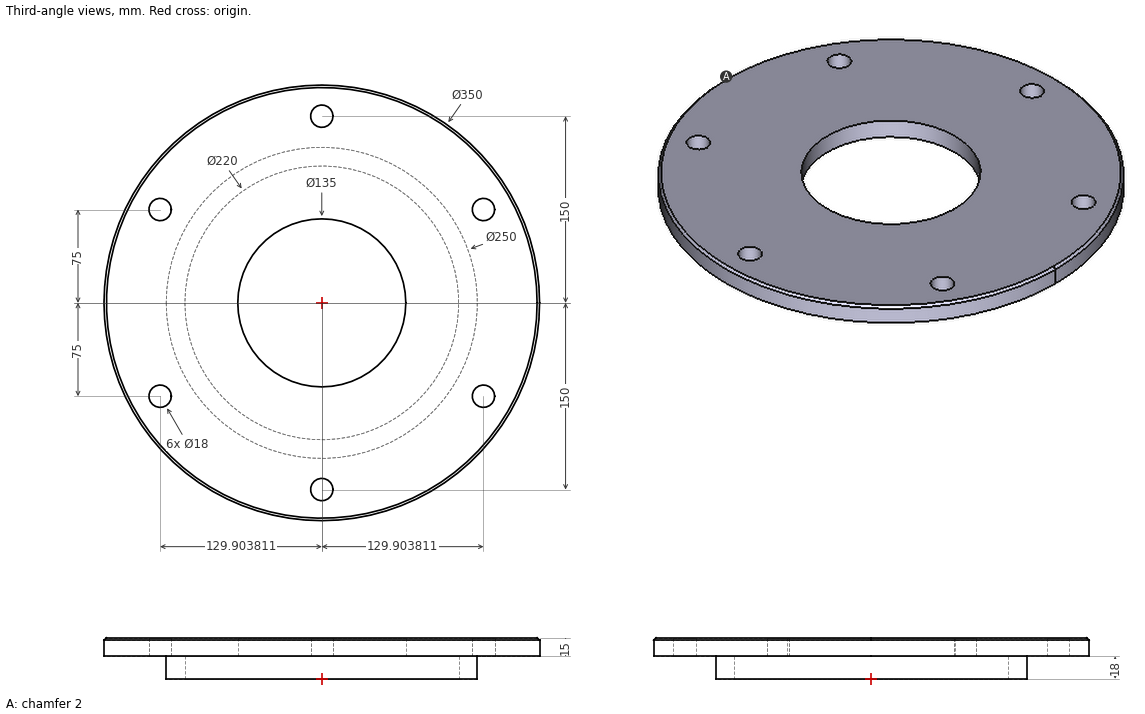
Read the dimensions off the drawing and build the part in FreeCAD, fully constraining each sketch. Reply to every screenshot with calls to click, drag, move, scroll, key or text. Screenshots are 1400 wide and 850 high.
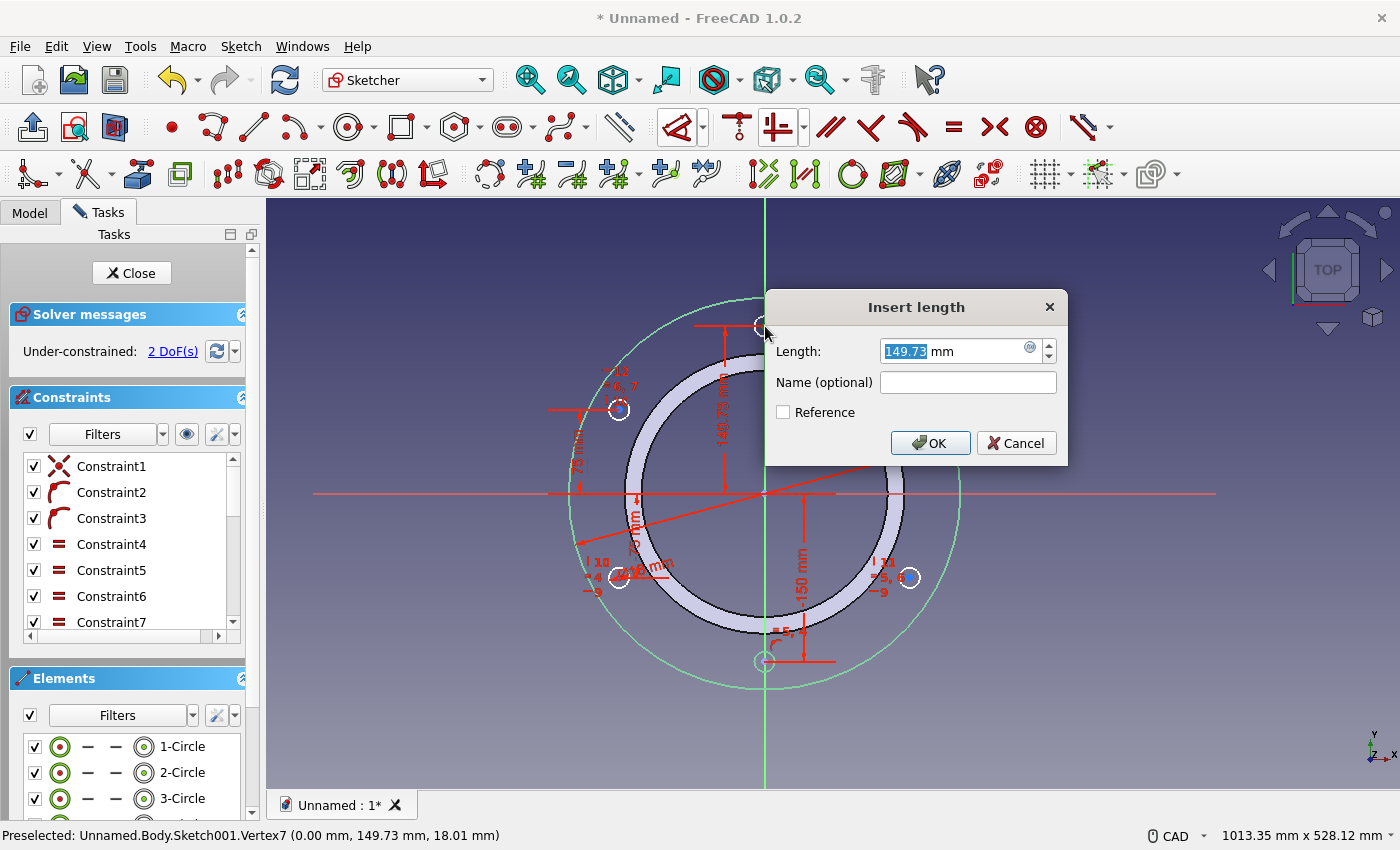
text(150)
key(Return)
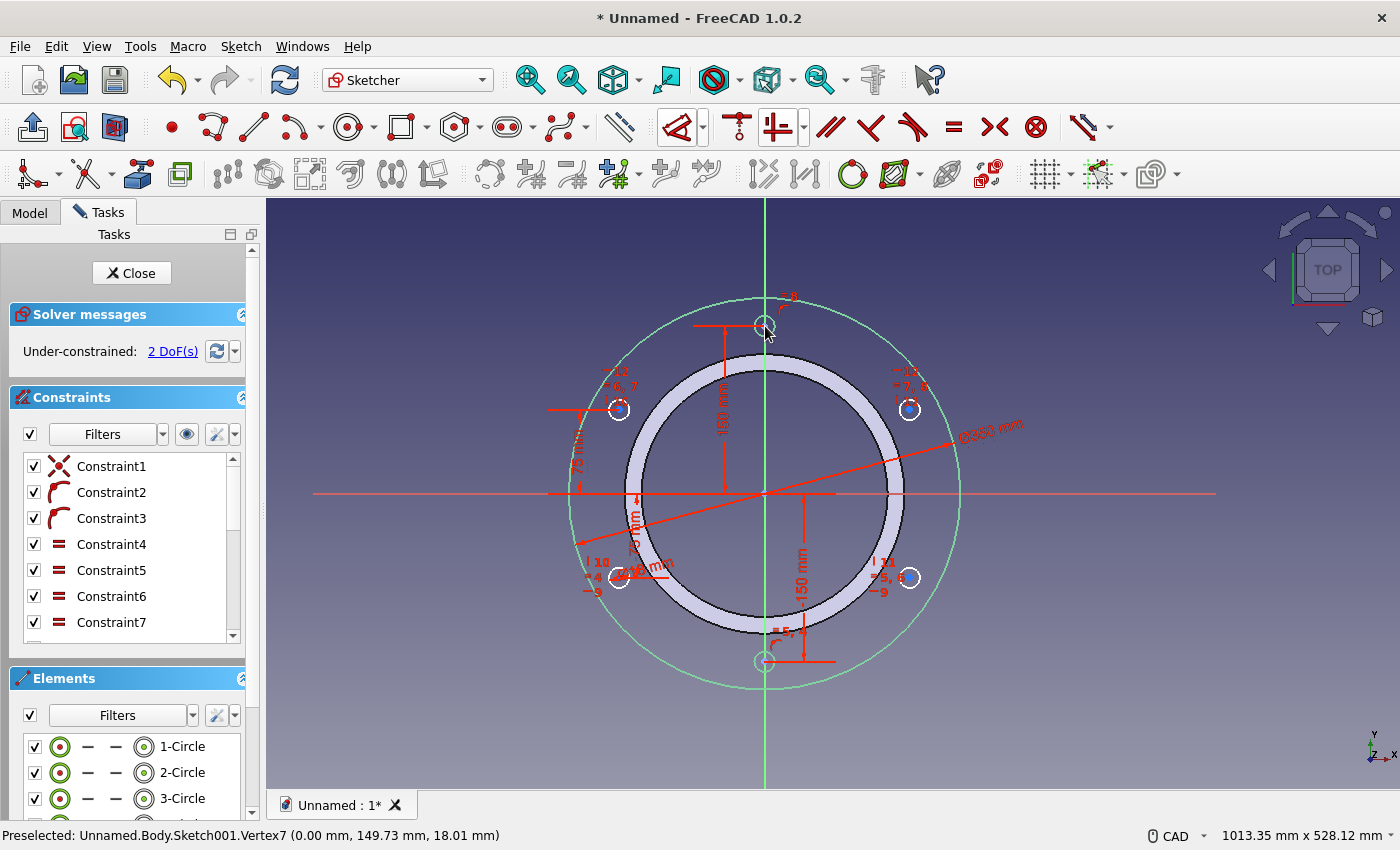
click(619, 578)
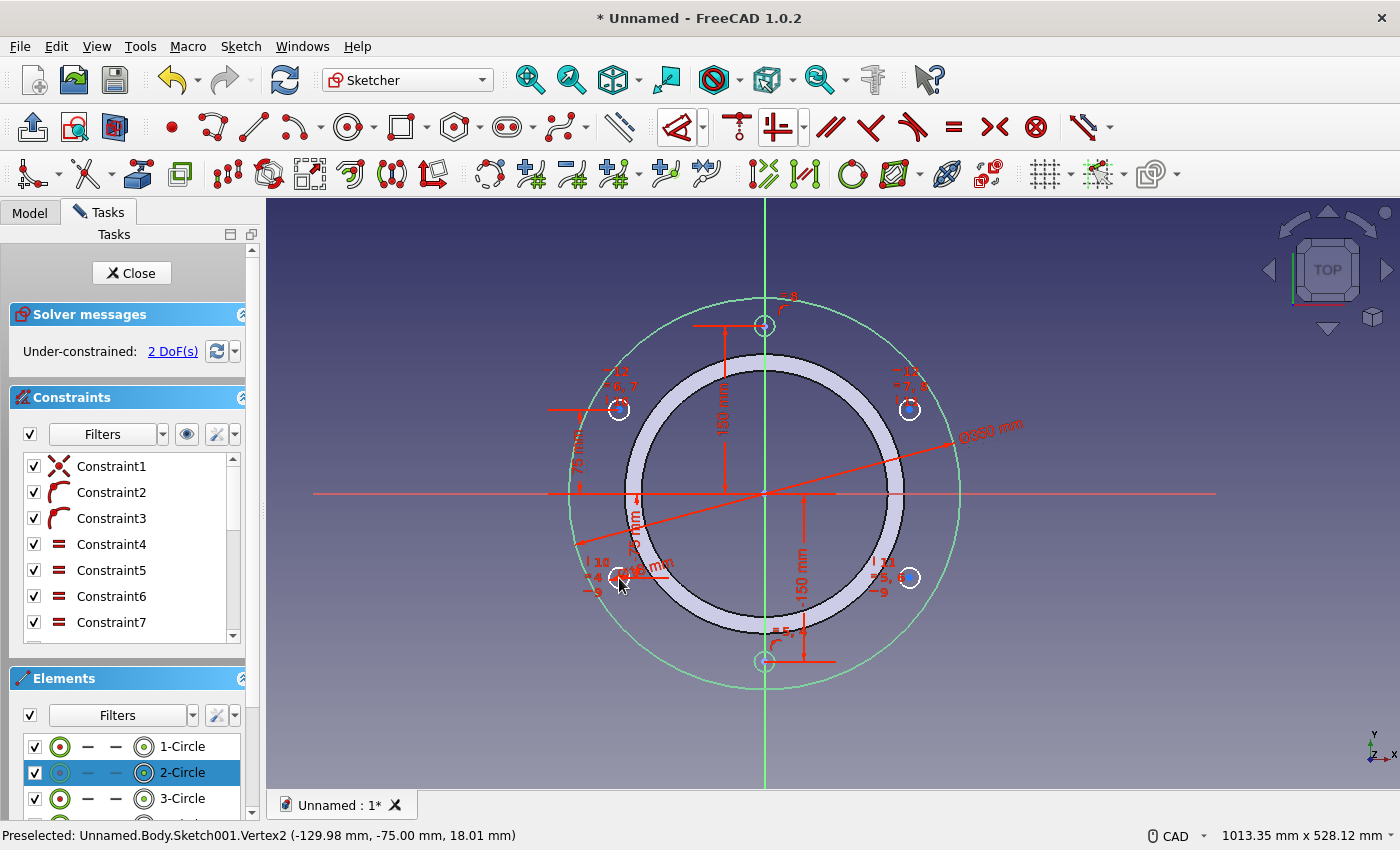
click(702, 128)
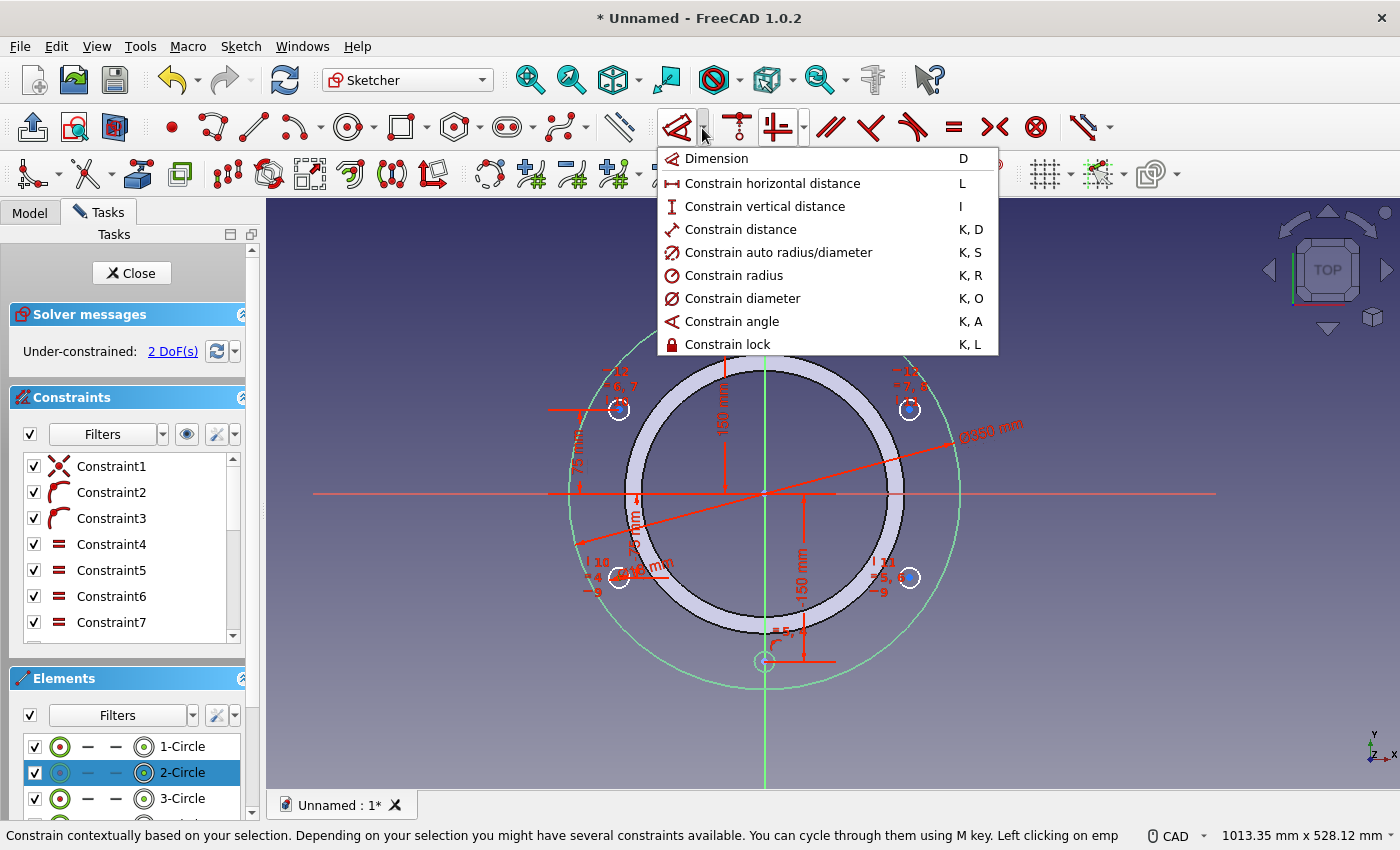
click(828, 184)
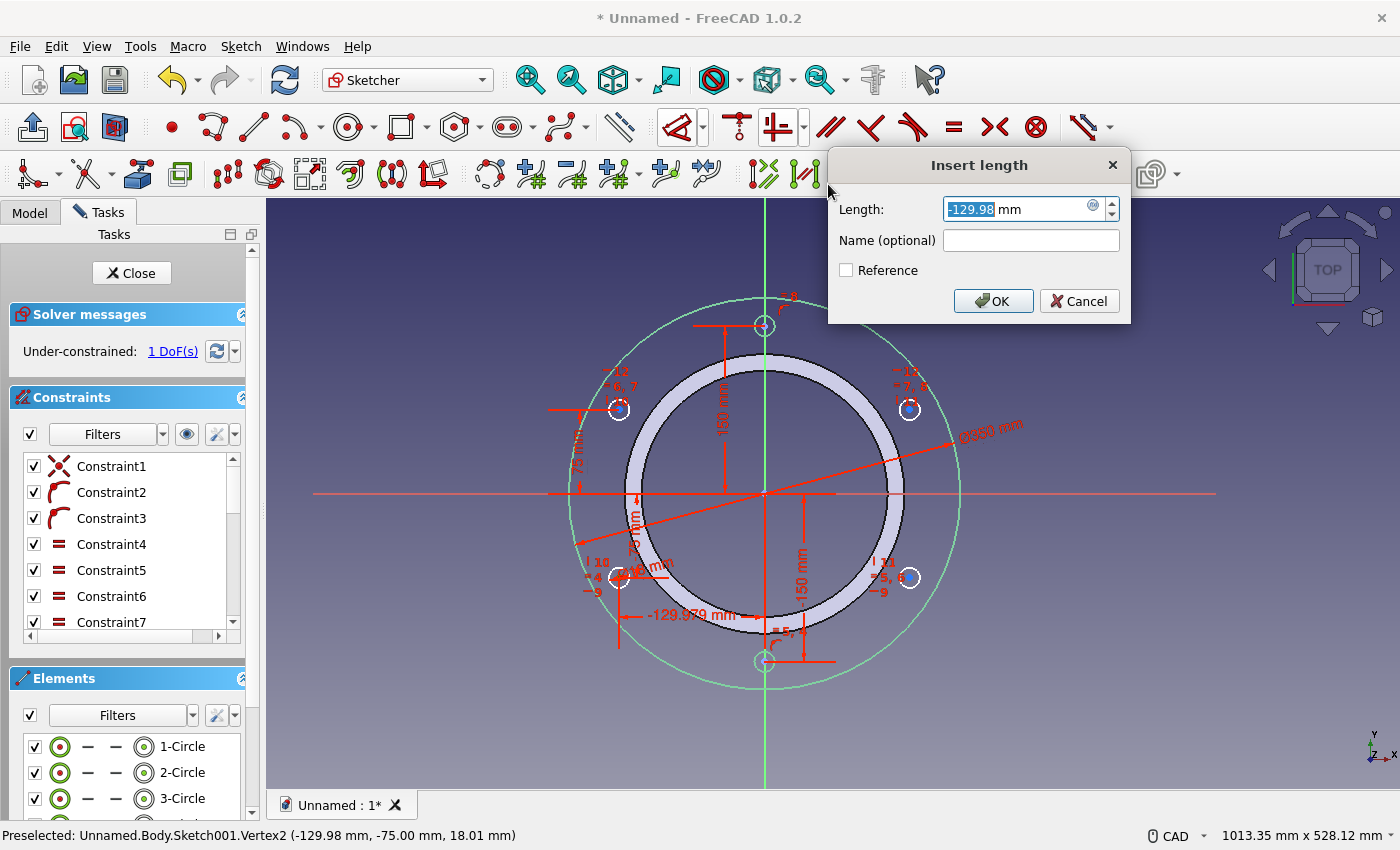
text(-129.903811)
key(Return)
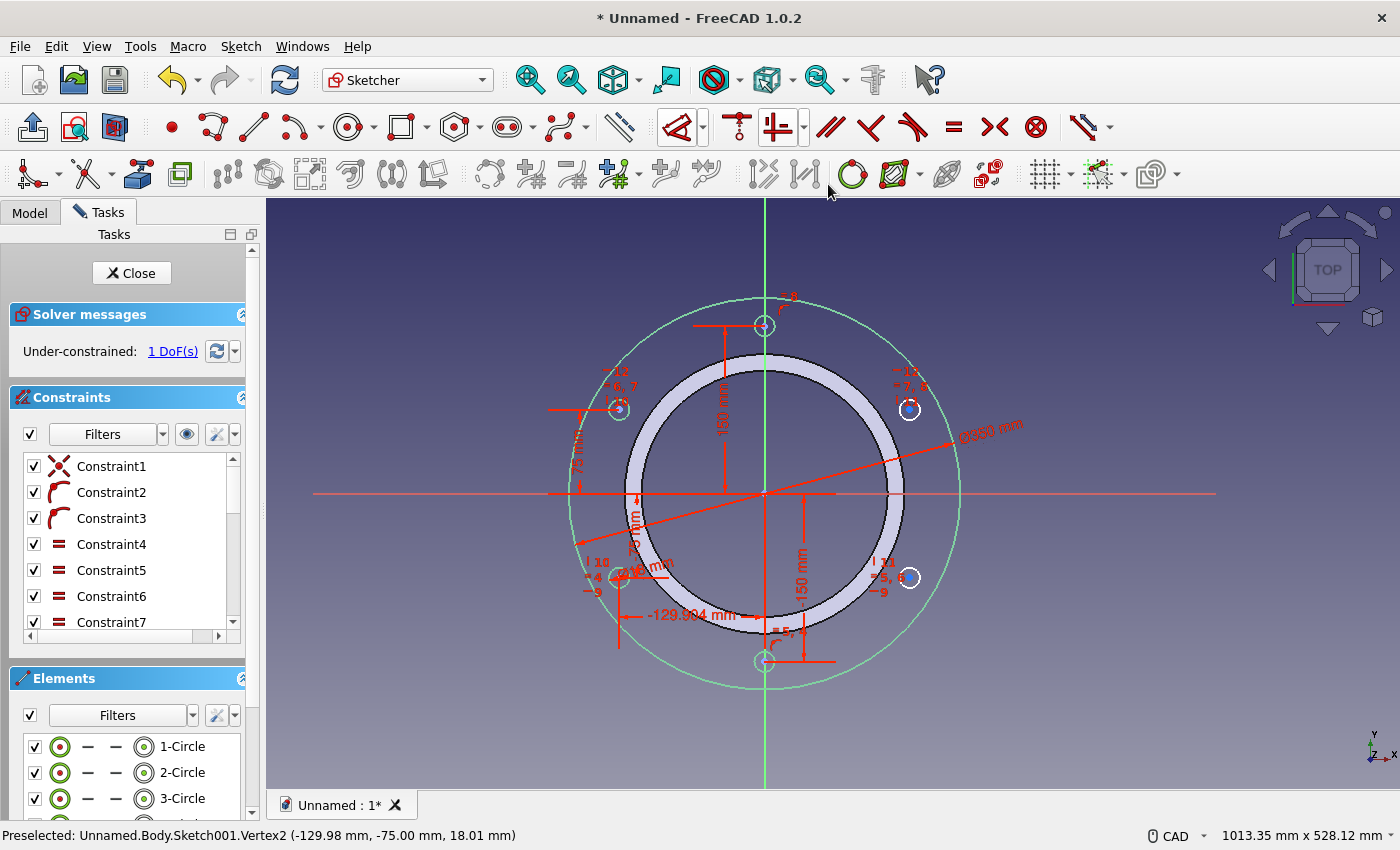
click(910, 578)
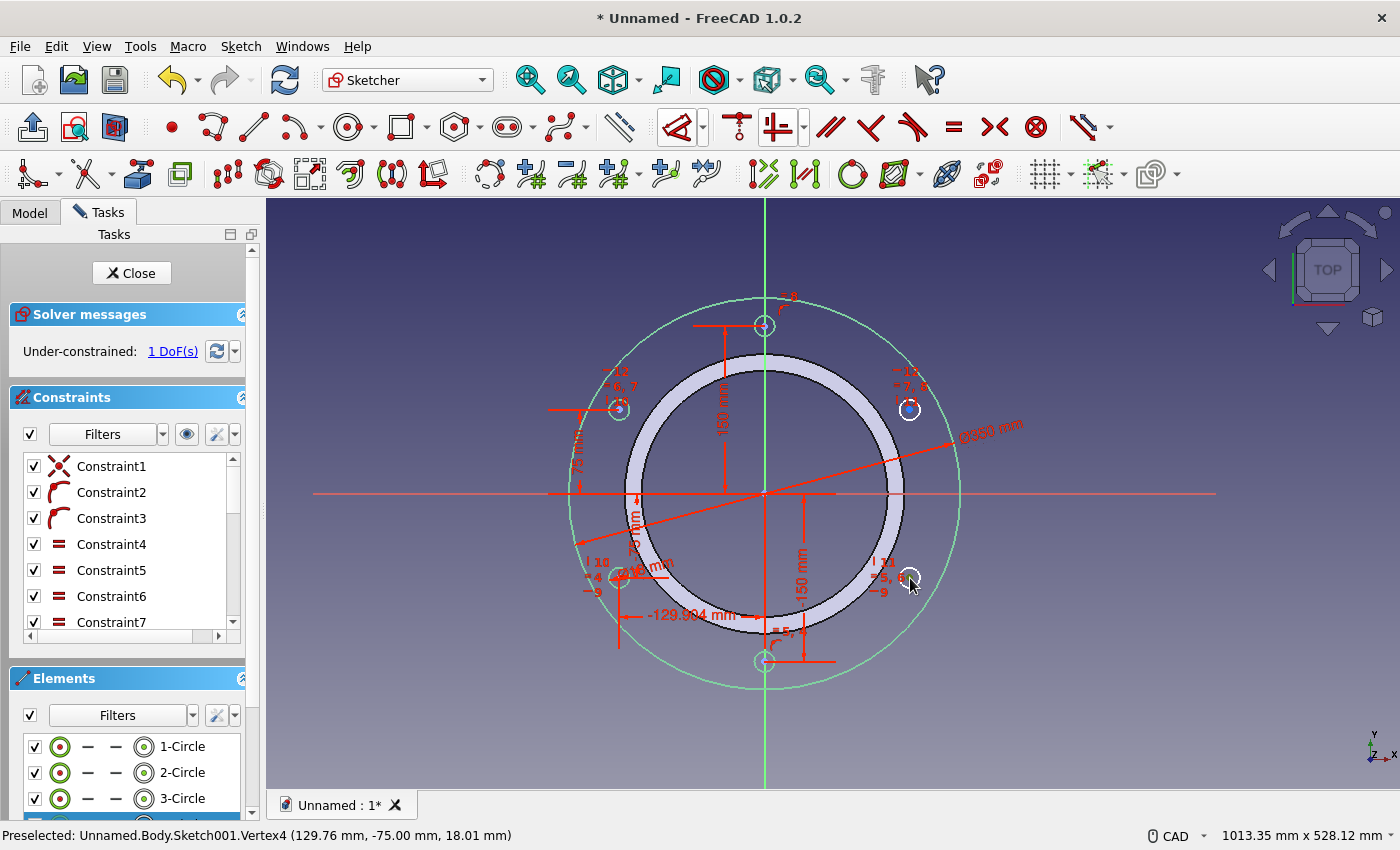
click(702, 128)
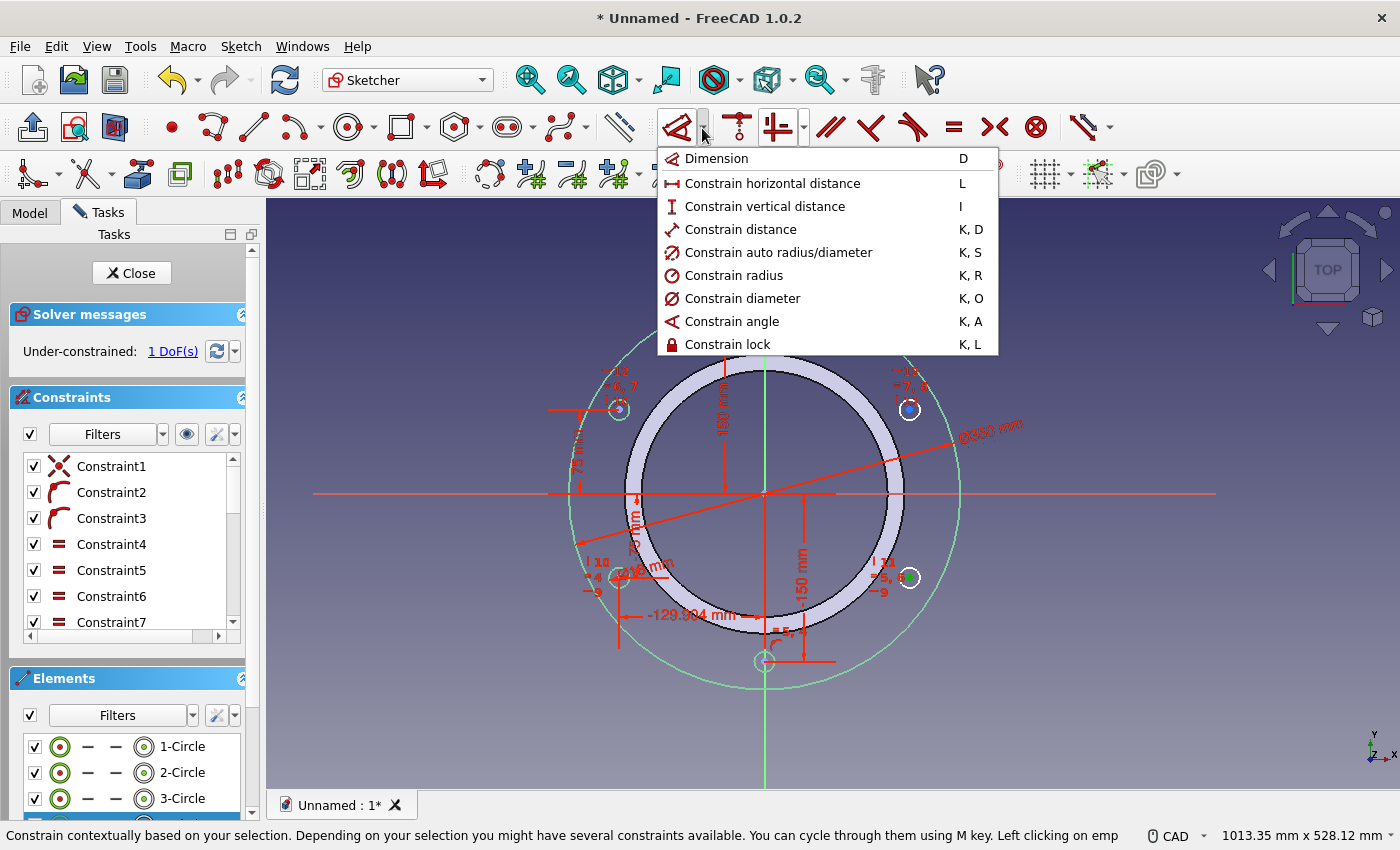
click(828, 184)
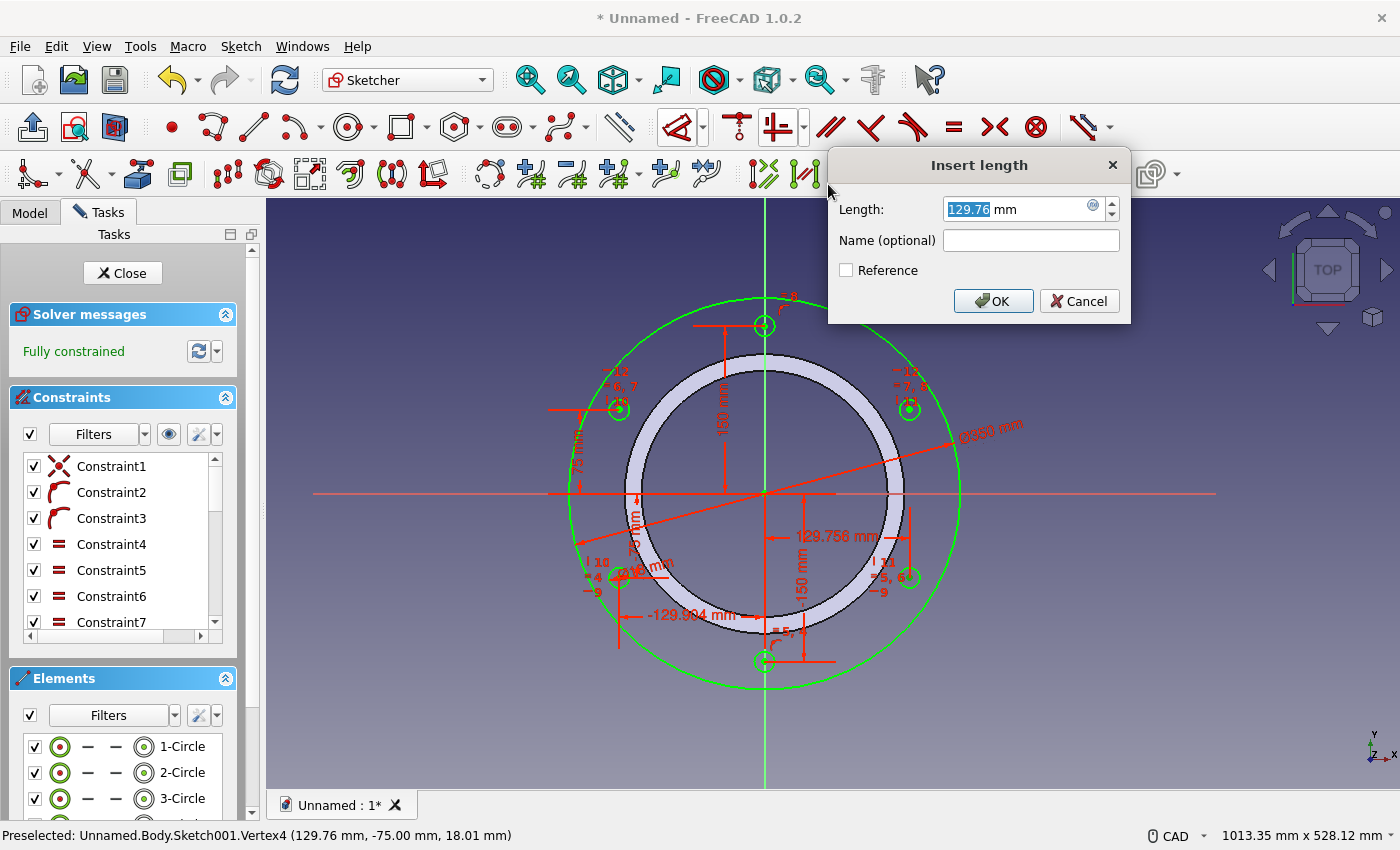
text(129.903811)
key(Return)